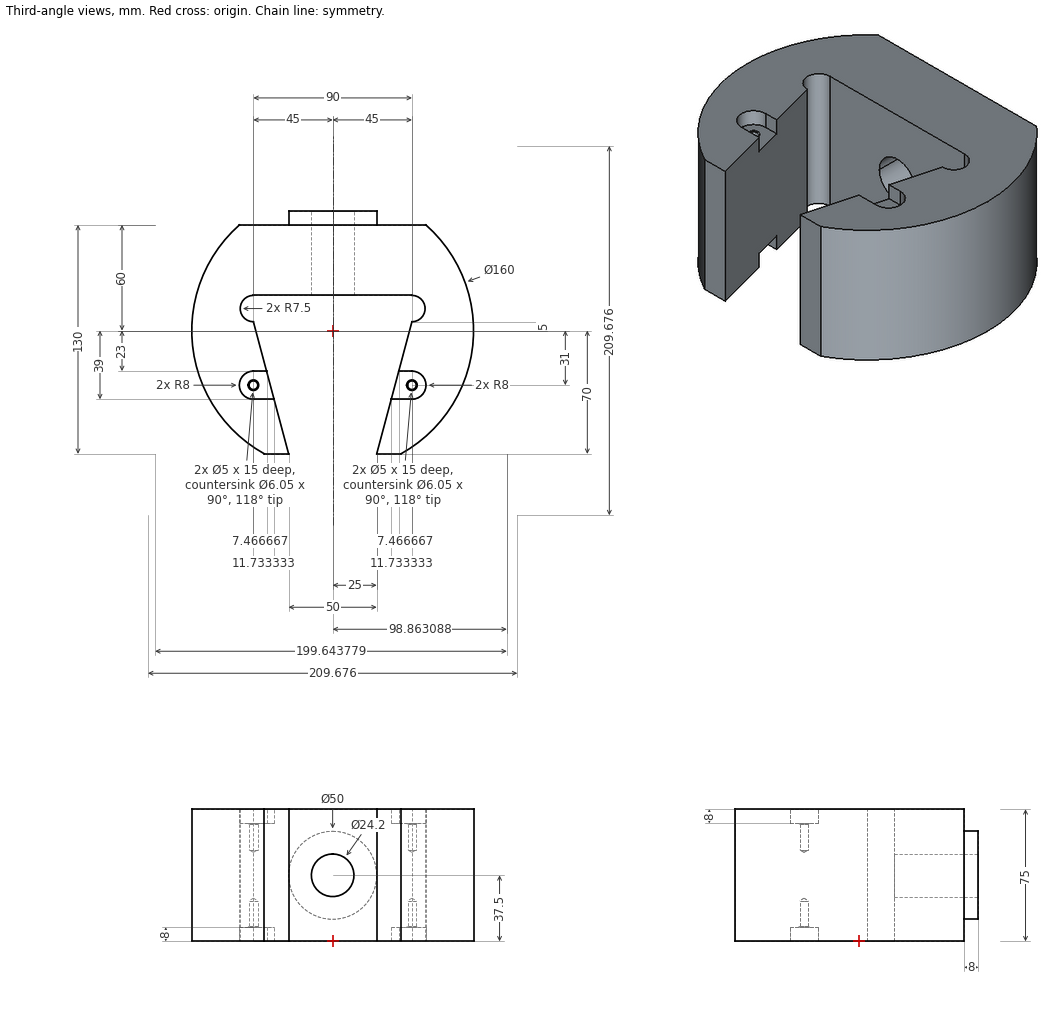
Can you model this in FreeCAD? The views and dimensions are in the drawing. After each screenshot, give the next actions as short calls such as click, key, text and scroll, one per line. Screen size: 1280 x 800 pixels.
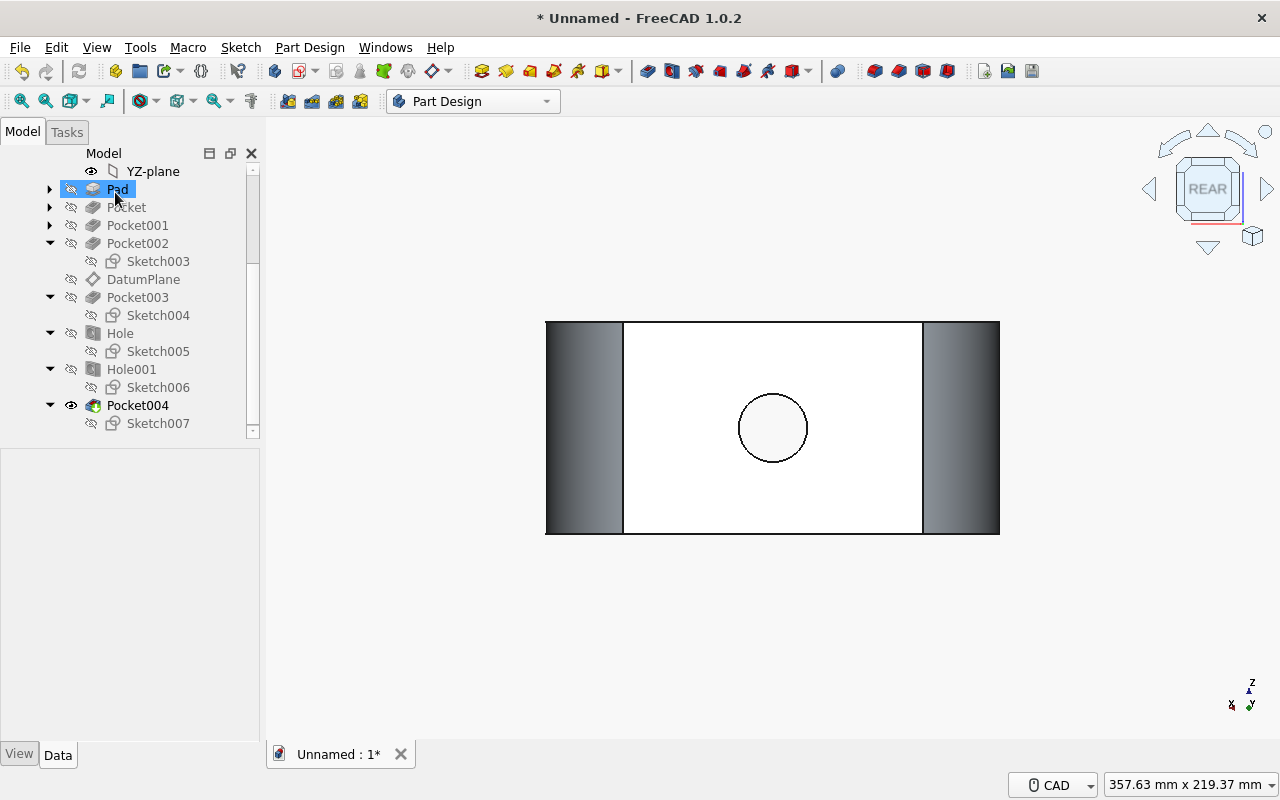
key(v)
key(f)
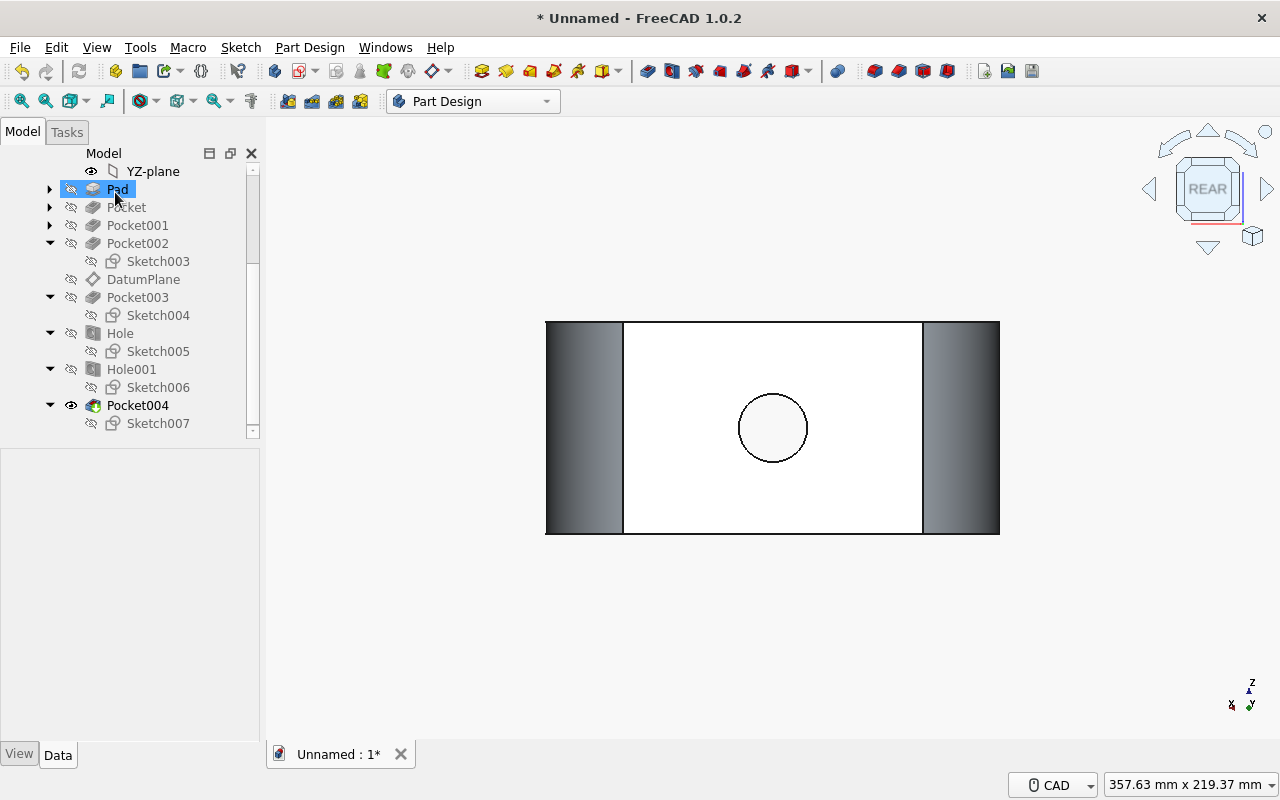
scroll(160, 293, down, 3)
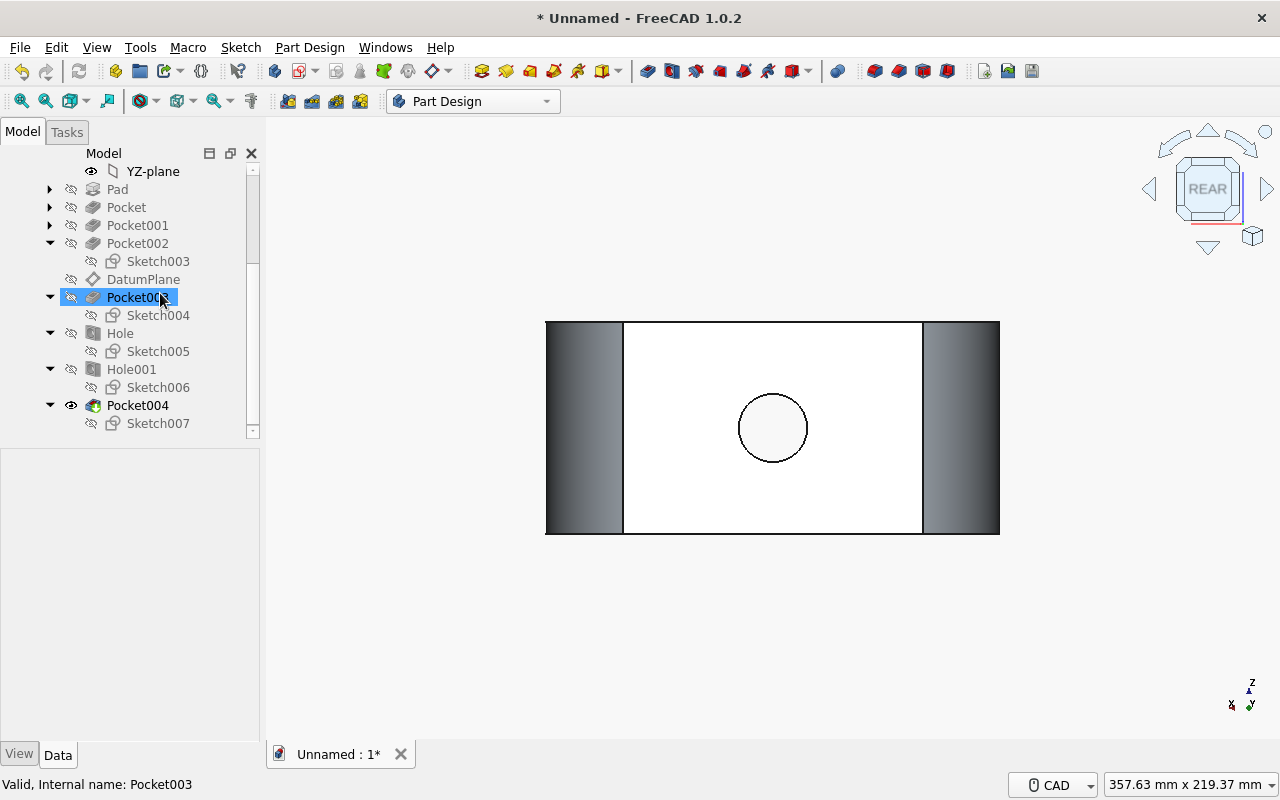
scroll(160, 293, up, 15)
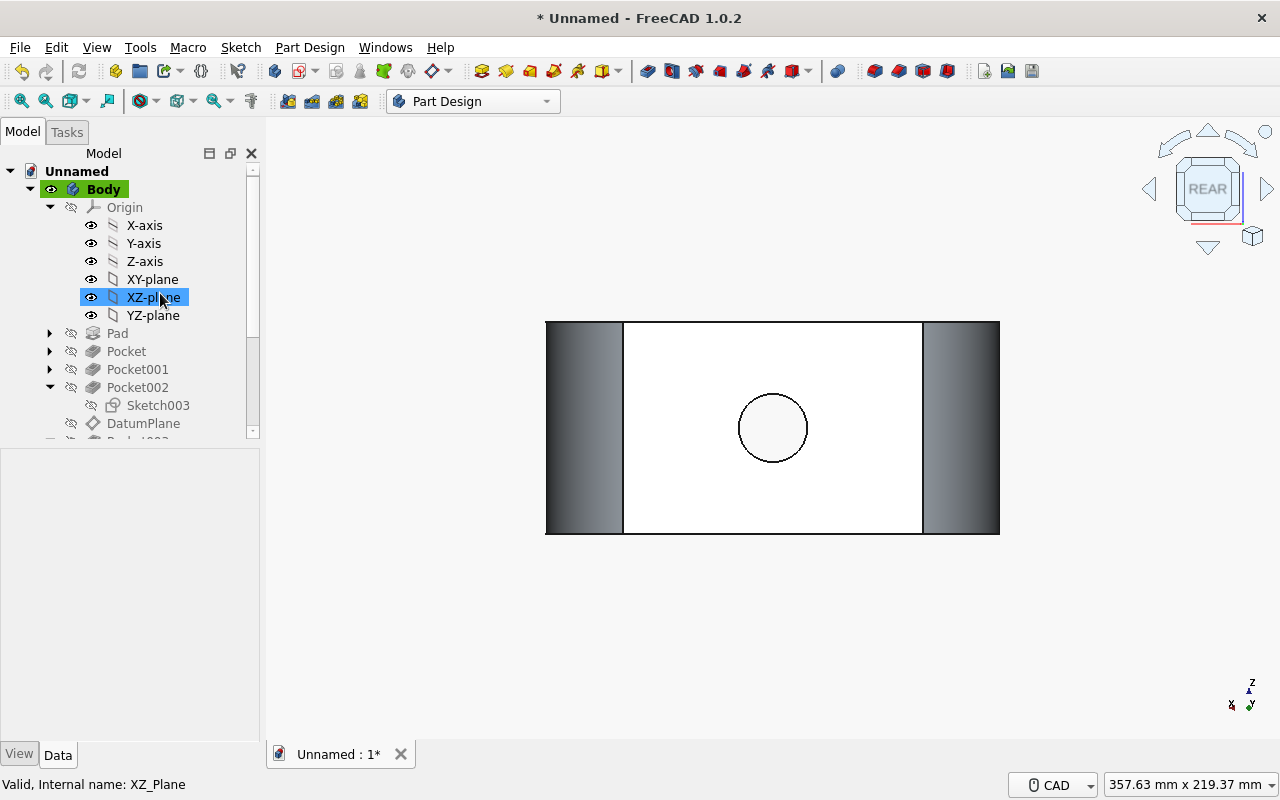
click(136, 297)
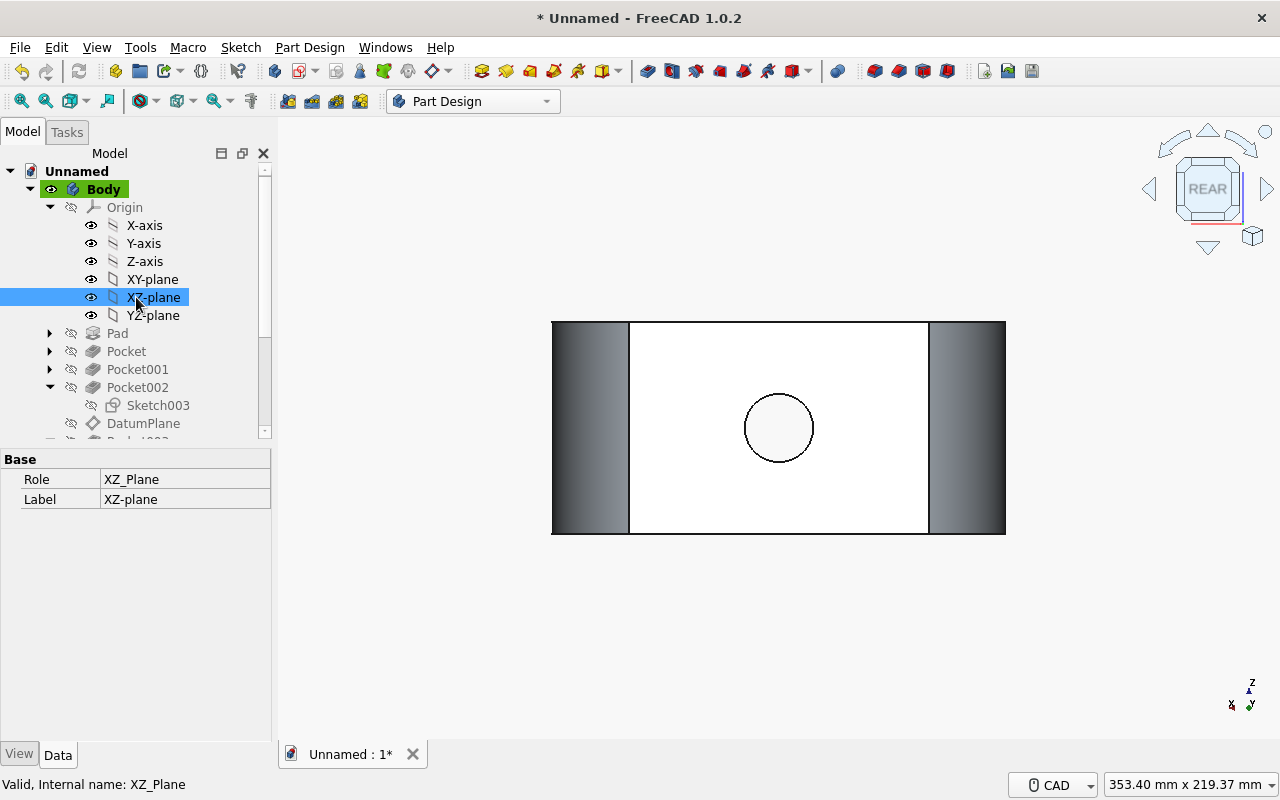
click(432, 72)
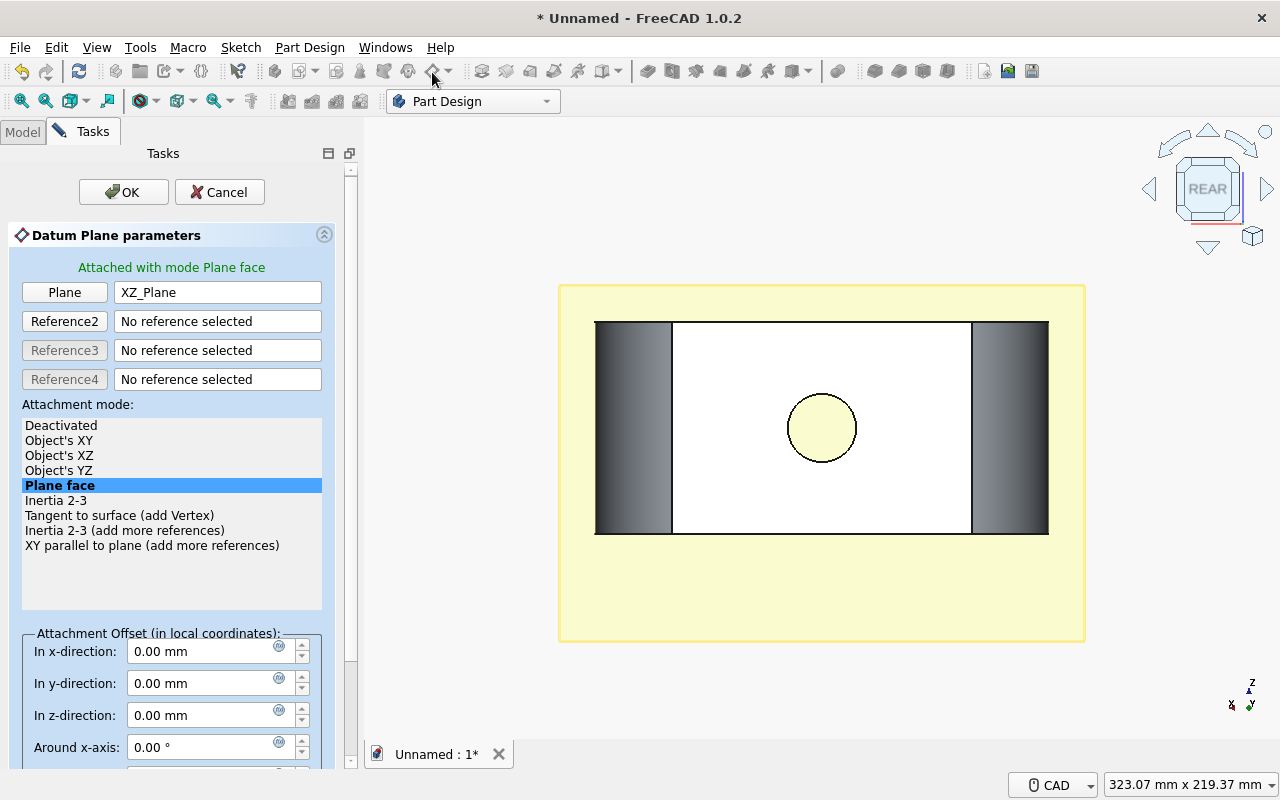
triple_click(210, 715)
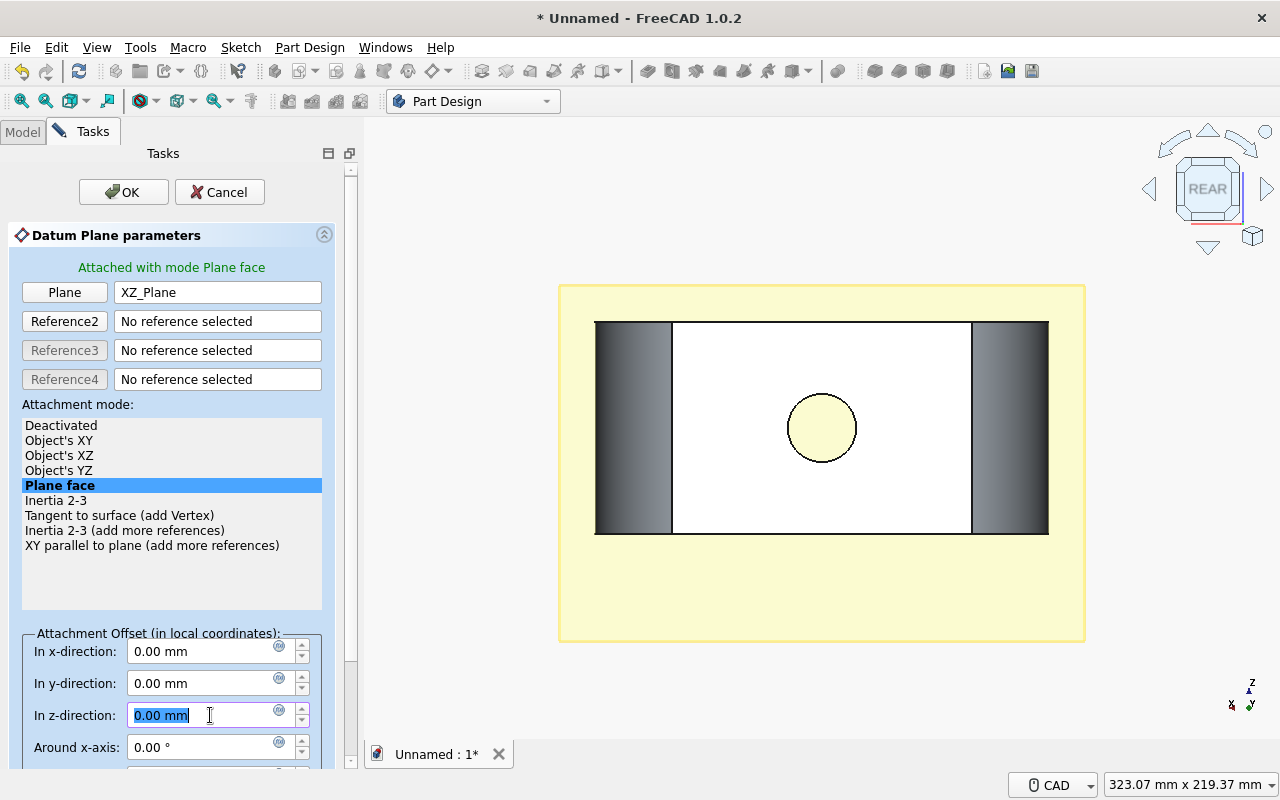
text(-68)
key(Tab)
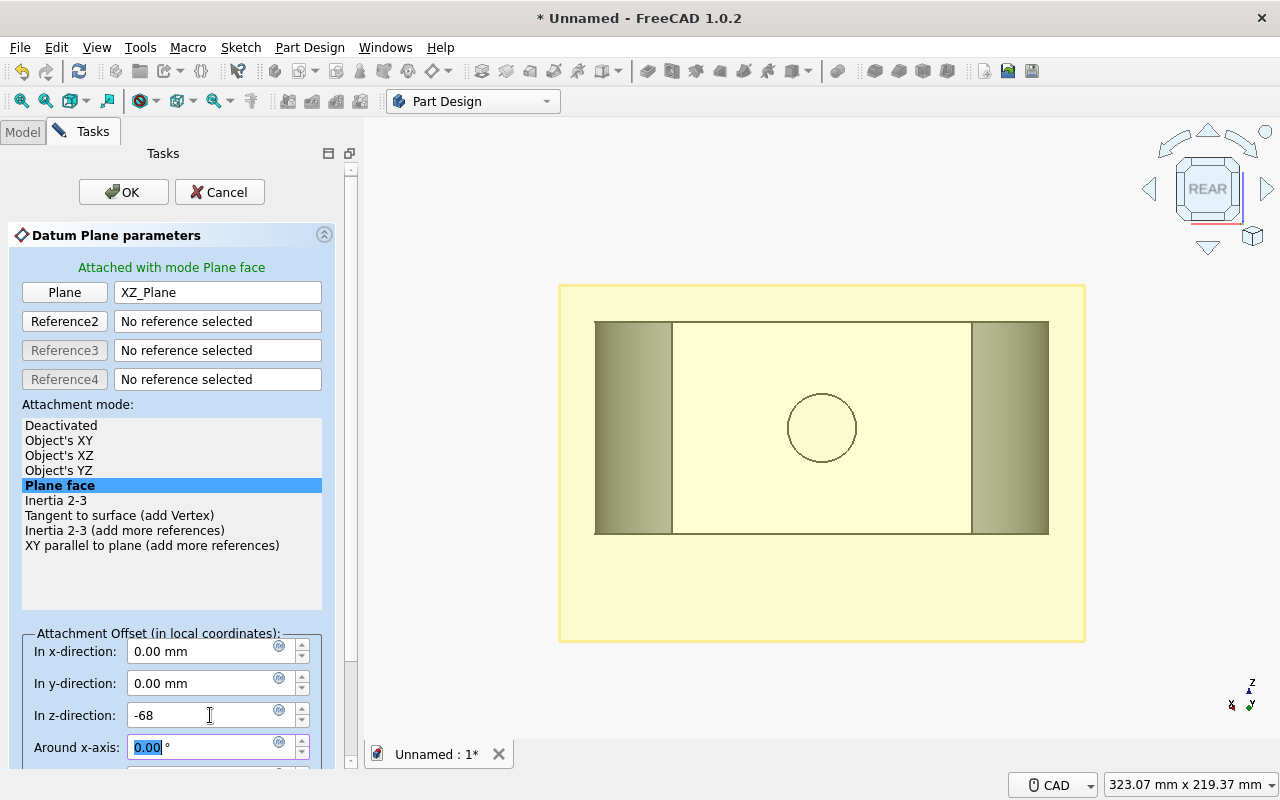
click(124, 192)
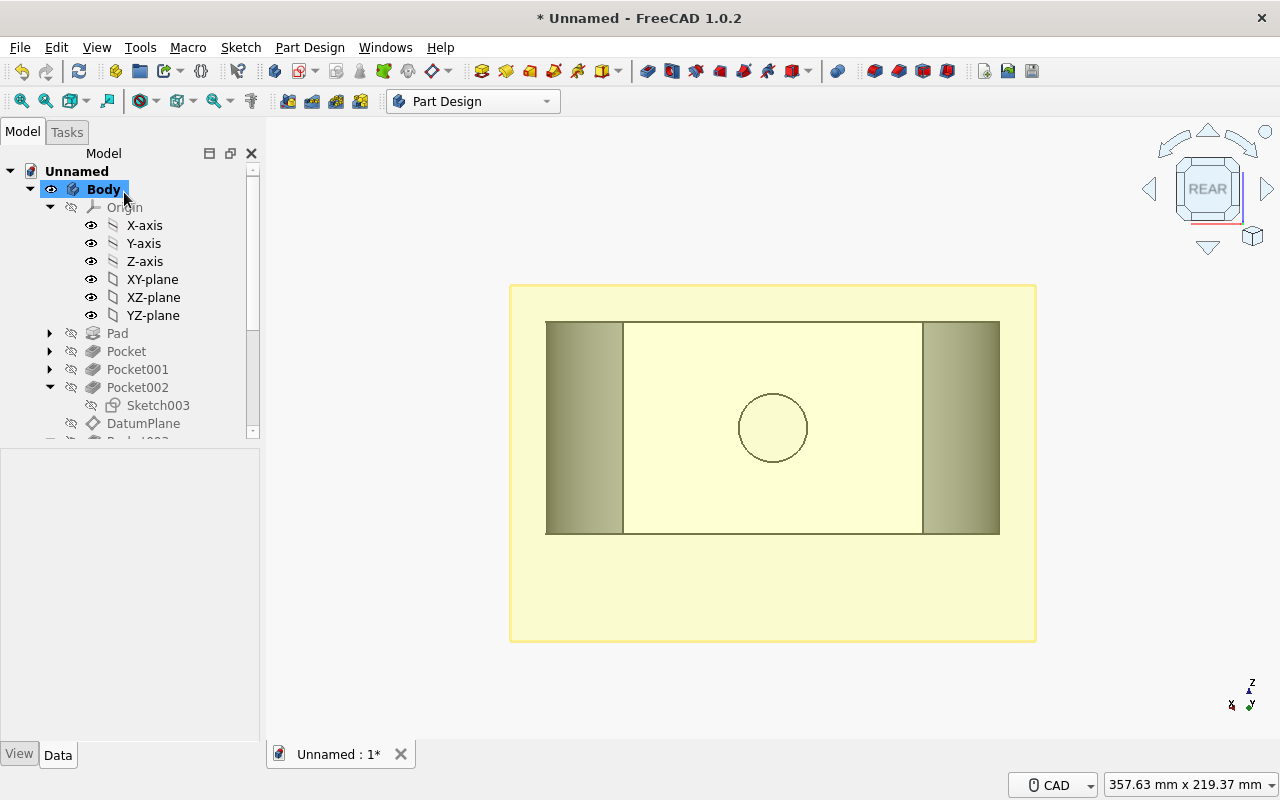
scroll(100, 293, down, 3)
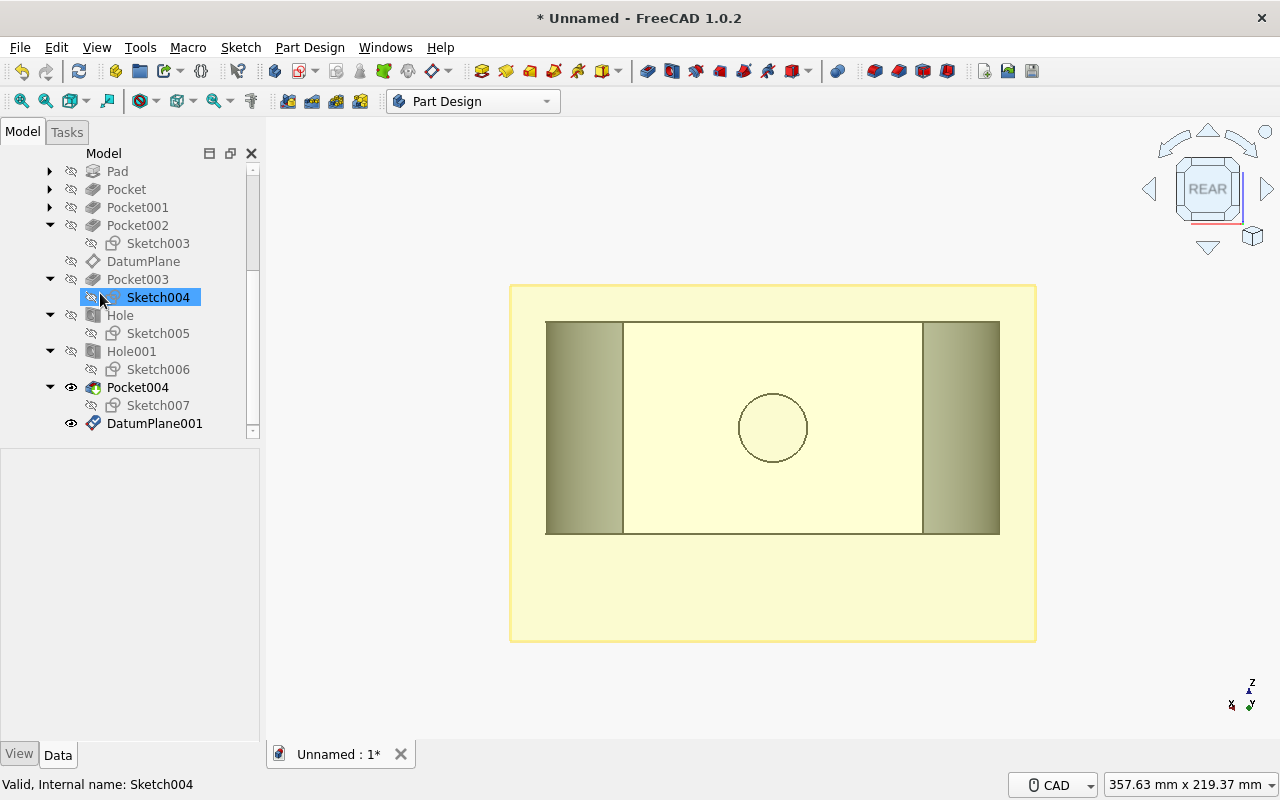
click(116, 423)